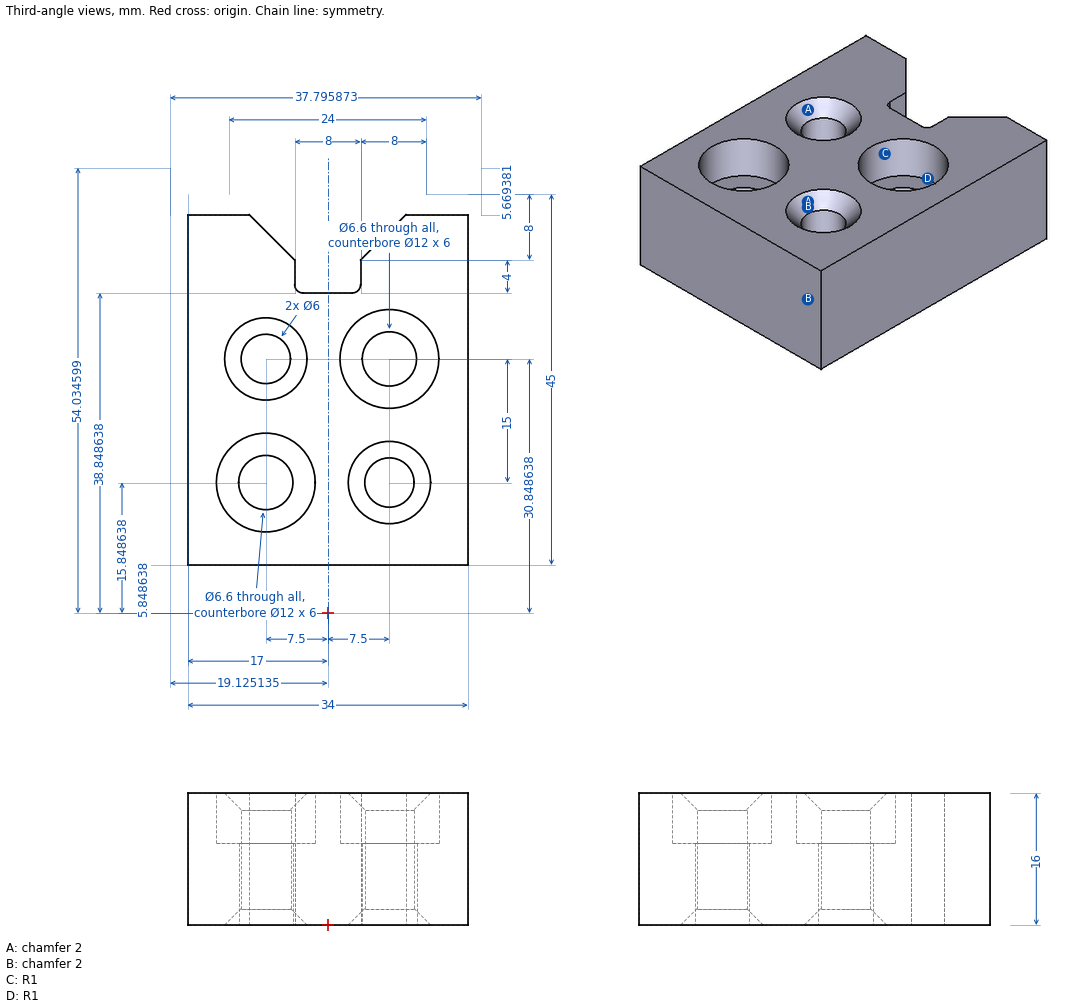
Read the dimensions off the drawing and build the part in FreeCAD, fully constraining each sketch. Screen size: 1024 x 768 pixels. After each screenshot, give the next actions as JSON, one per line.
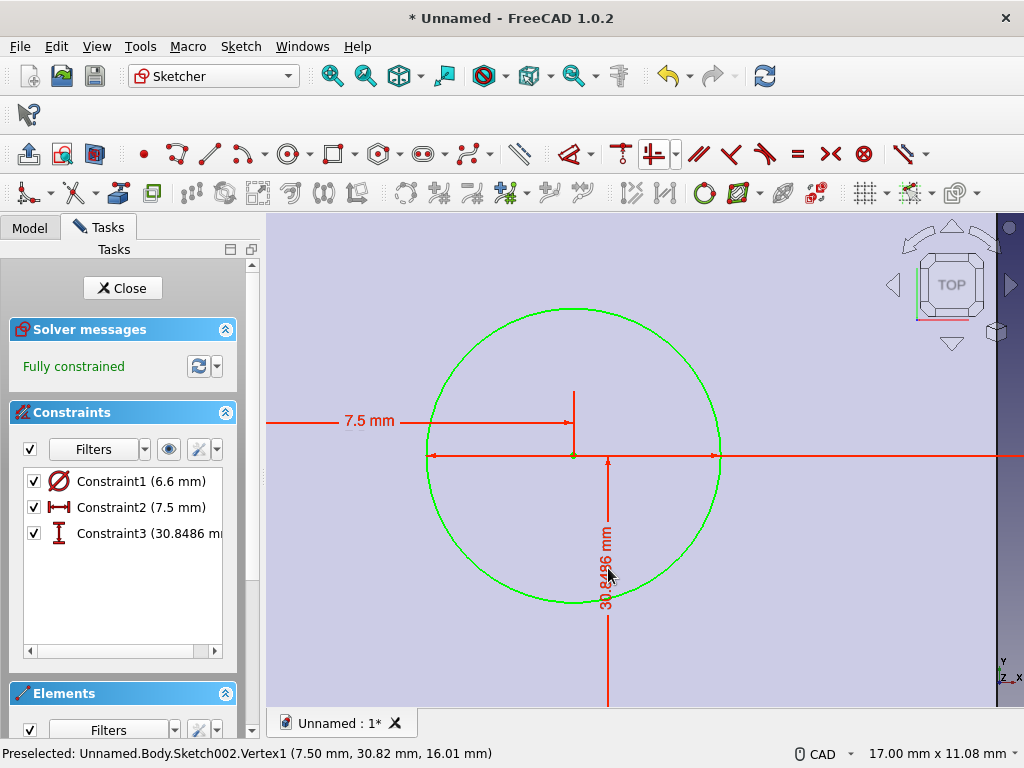
{"action": "left_click", "coordinate": [123, 288]}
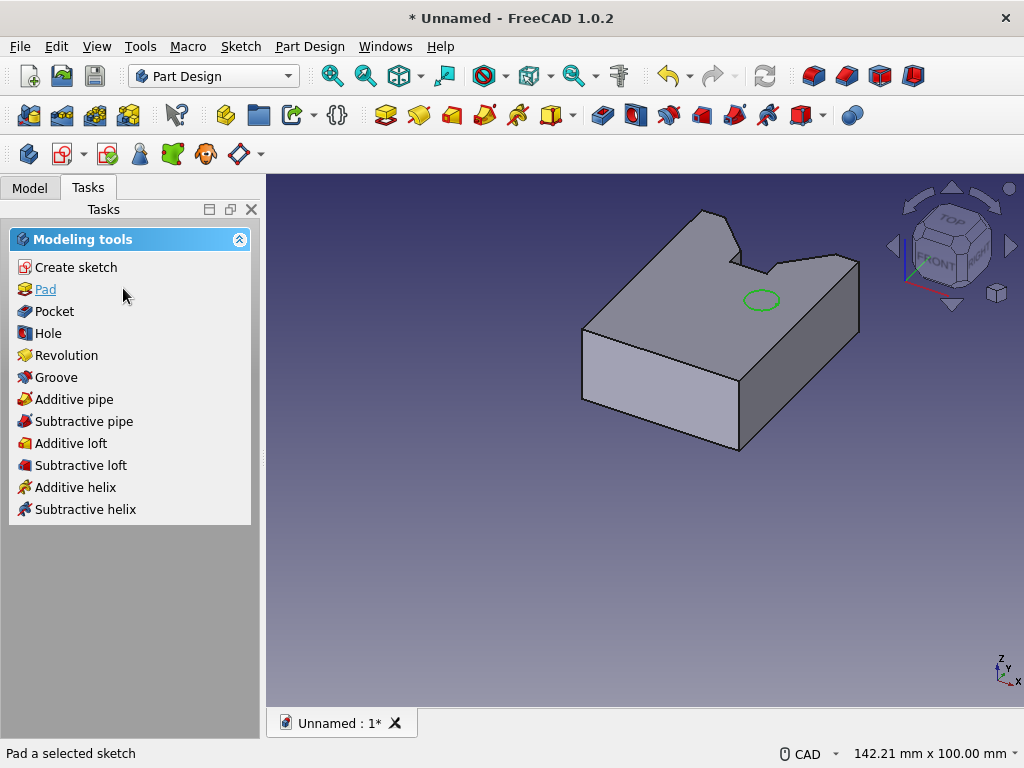
{"action": "left_click", "coordinate": [636, 116]}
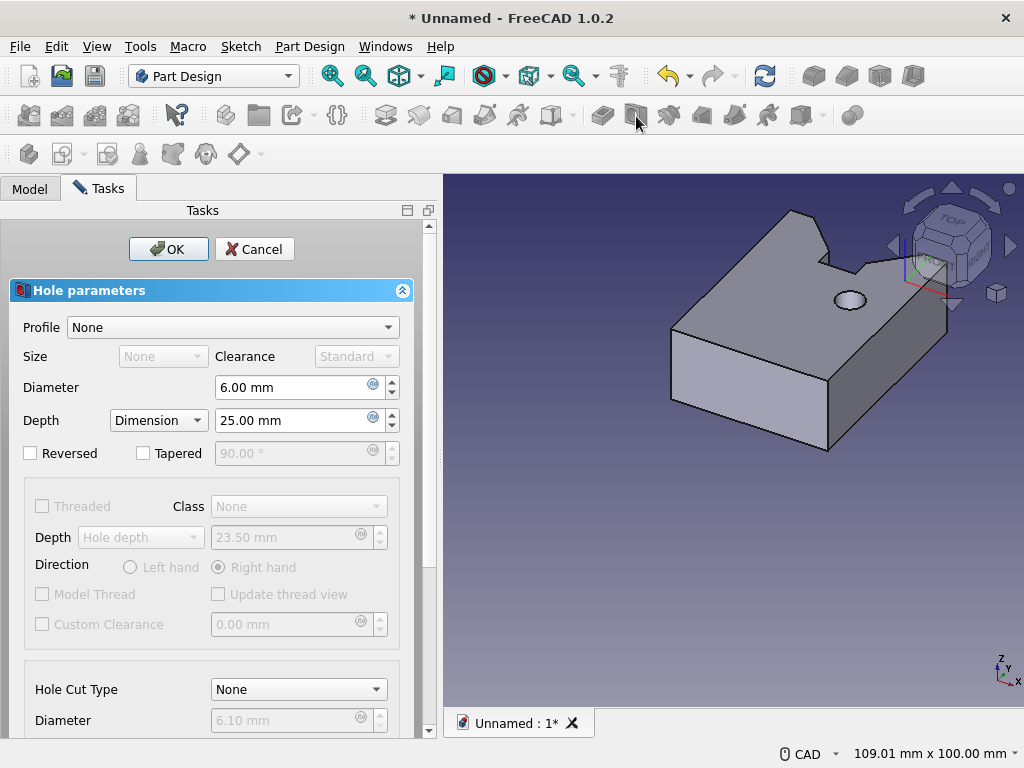
{"action": "triple_click", "coordinate": [300, 388]}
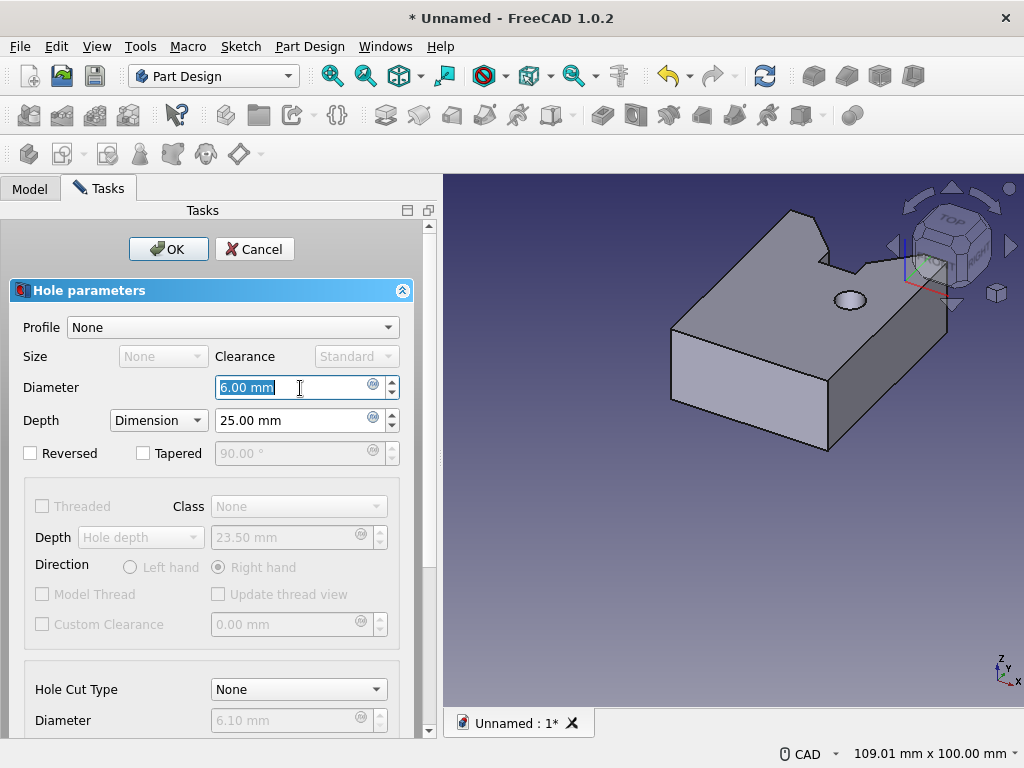
{"action": "type", "text": "6.6"}
{"action": "key", "text": "Tab"}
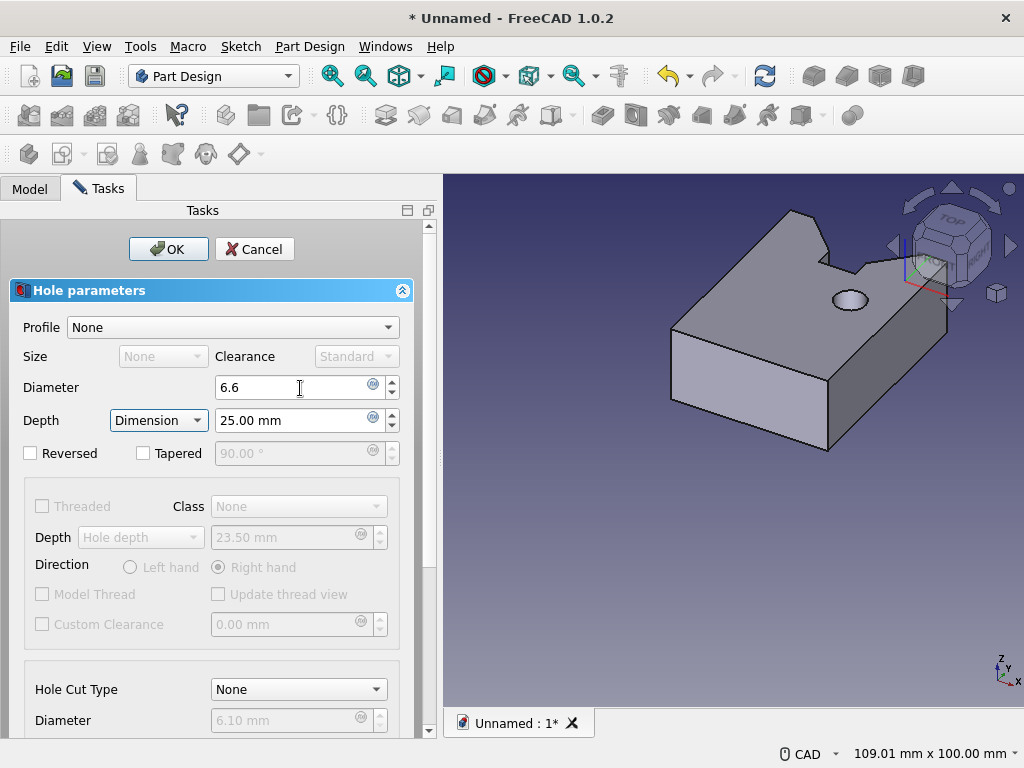
{"action": "left_click", "coordinate": [160, 420]}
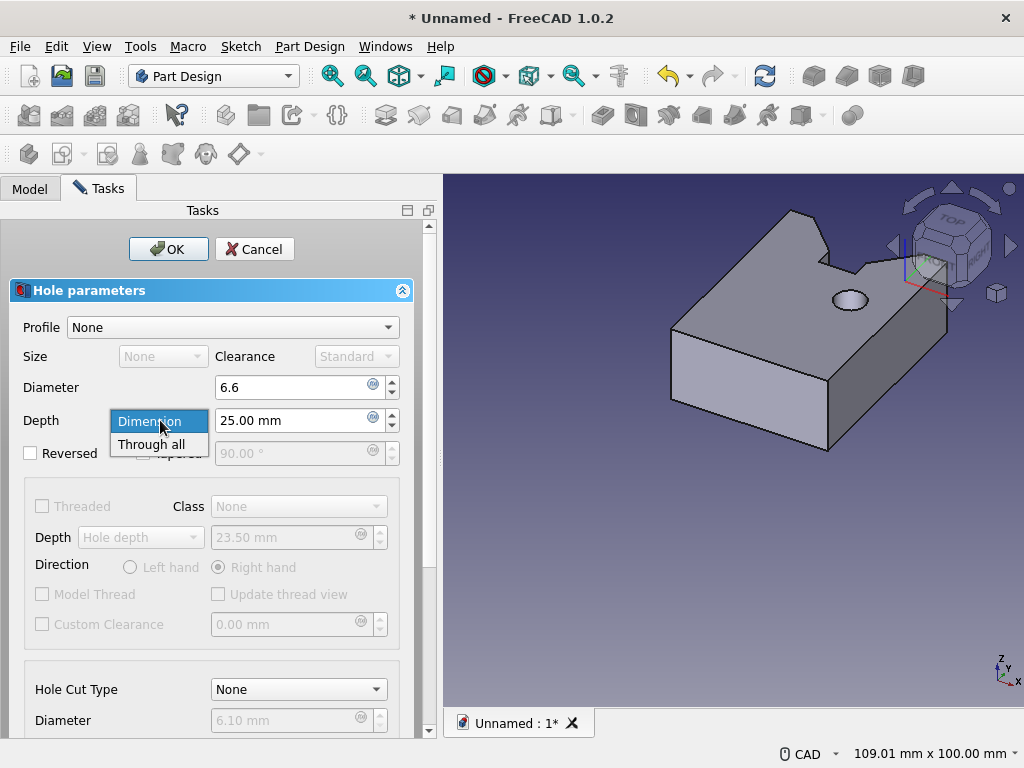
{"action": "left_click", "coordinate": [158, 444]}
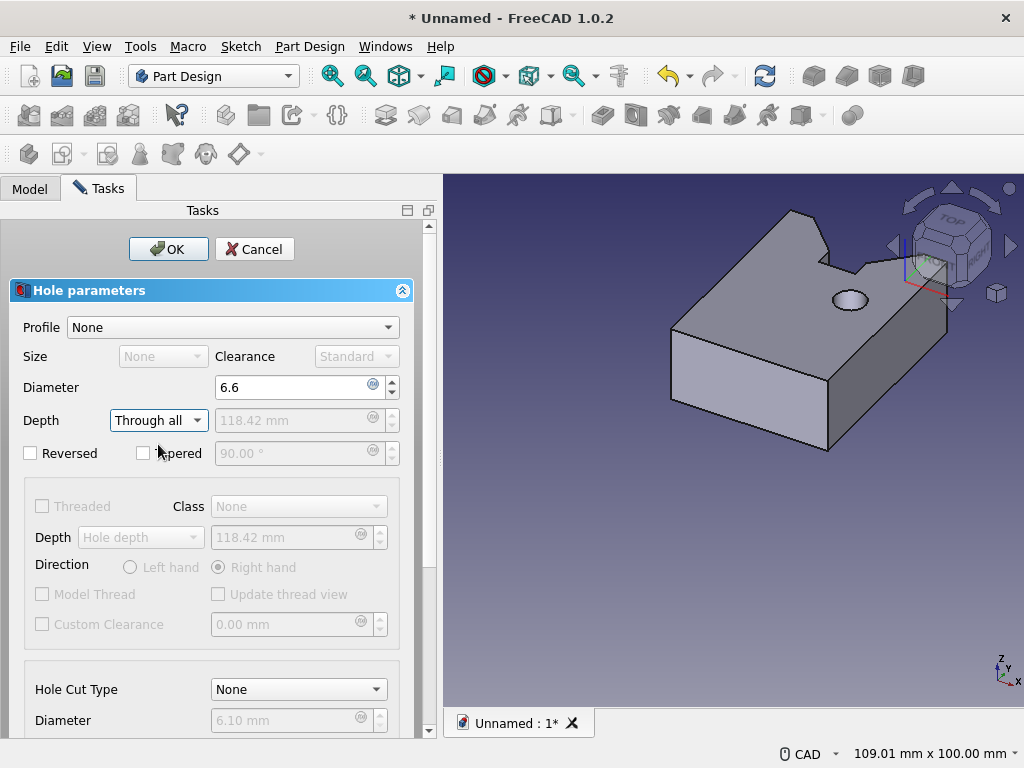
{"action": "left_click", "coordinate": [300, 690]}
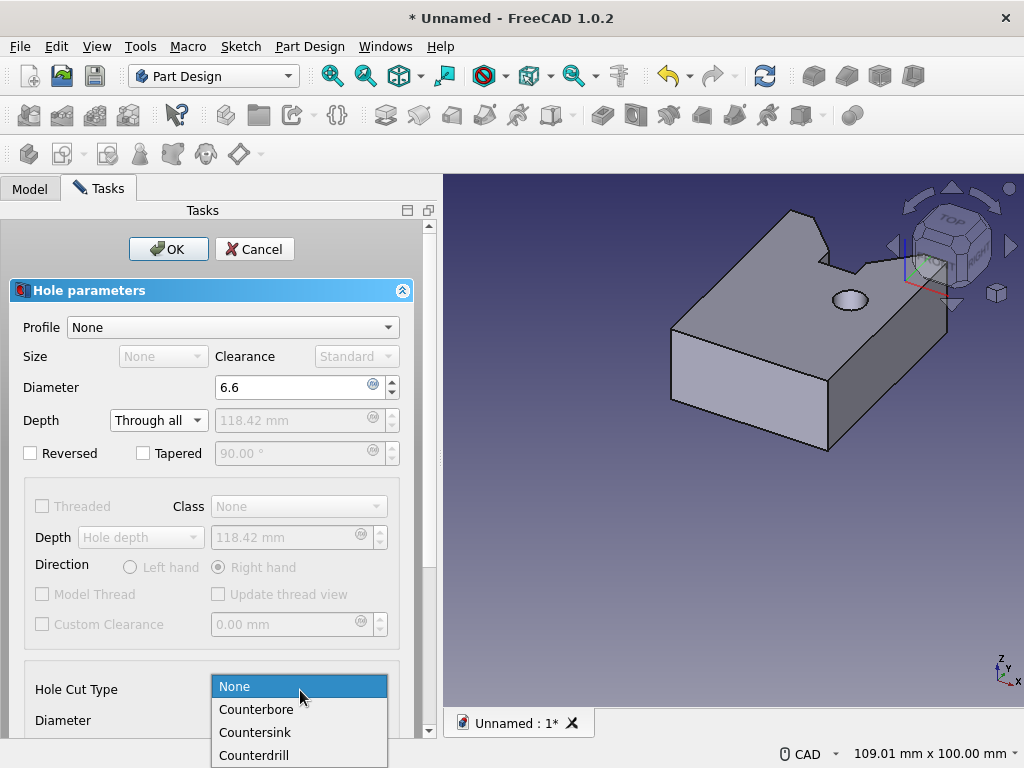
{"action": "left_click", "coordinate": [298, 710]}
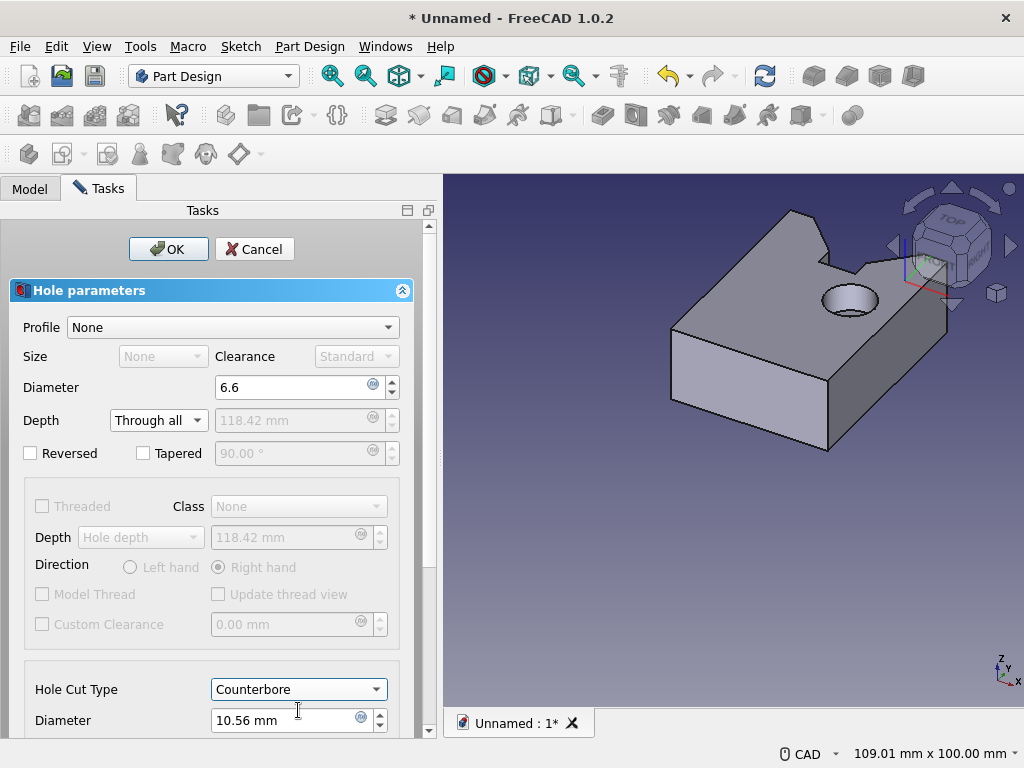
{"action": "triple_click", "coordinate": [292, 720]}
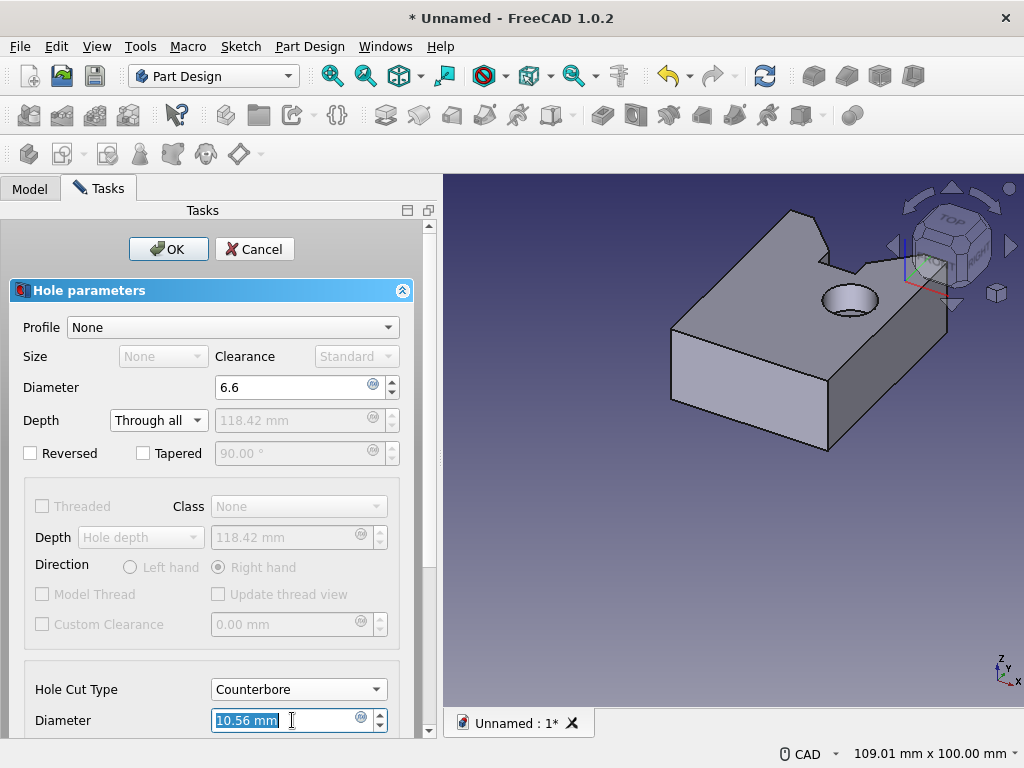
{"action": "type", "text": "12"}
{"action": "key", "text": "Tab"}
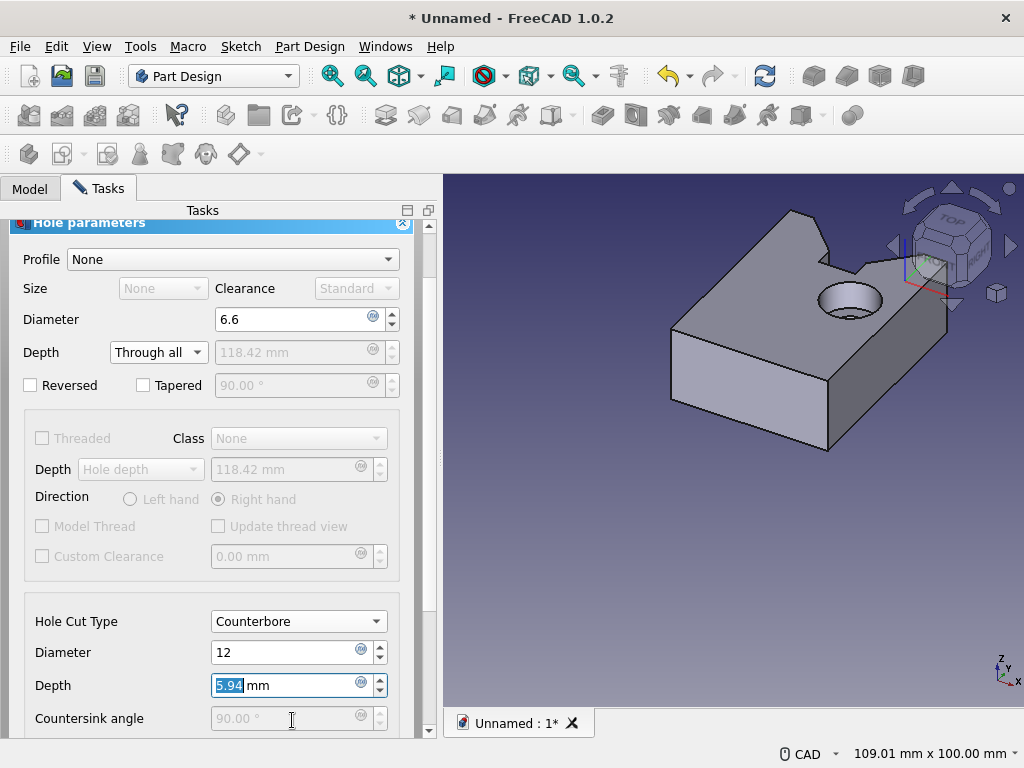
{"action": "type", "text": "6"}
{"action": "key", "text": "Tab"}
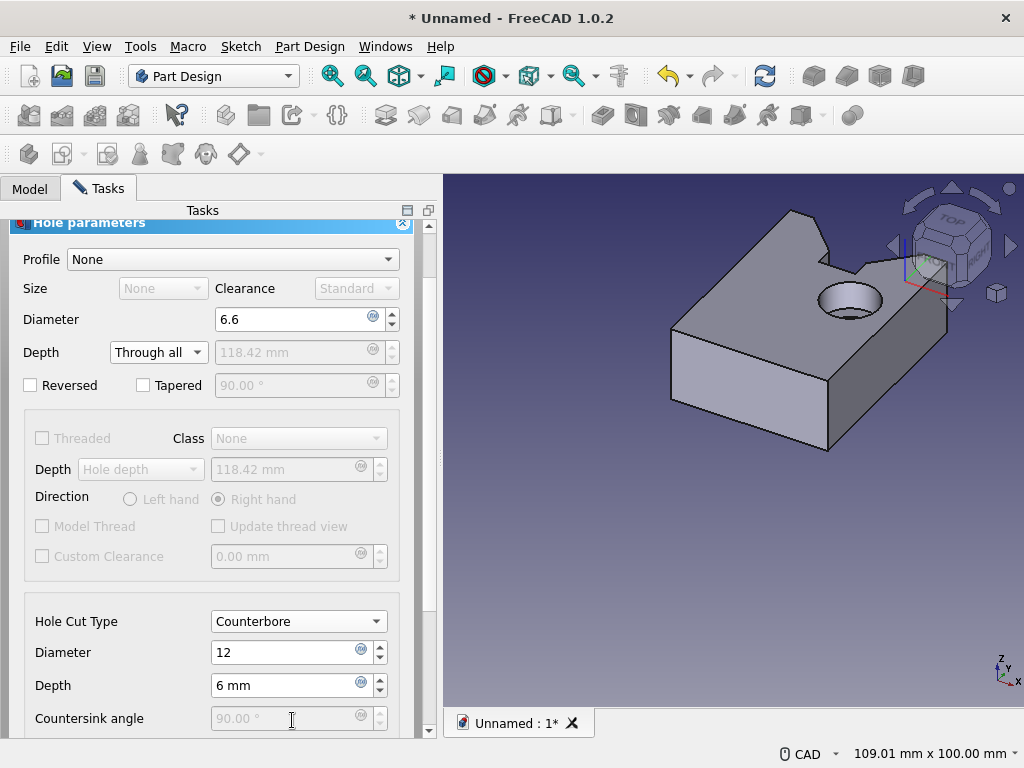
{"action": "scroll", "coordinate": [429, 479], "scroll_direction": "up", "scroll_amount": 2}